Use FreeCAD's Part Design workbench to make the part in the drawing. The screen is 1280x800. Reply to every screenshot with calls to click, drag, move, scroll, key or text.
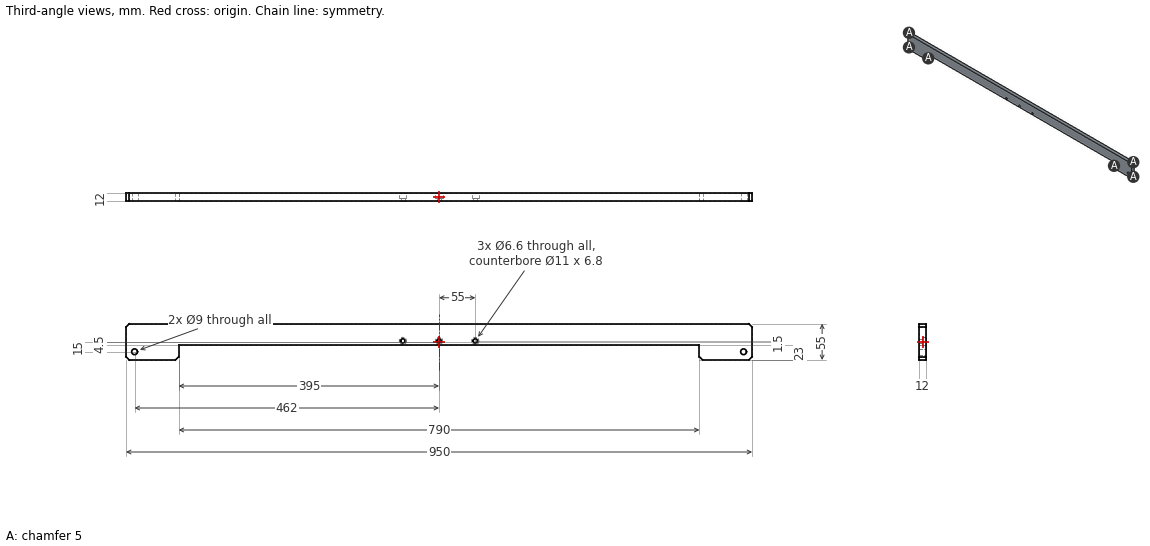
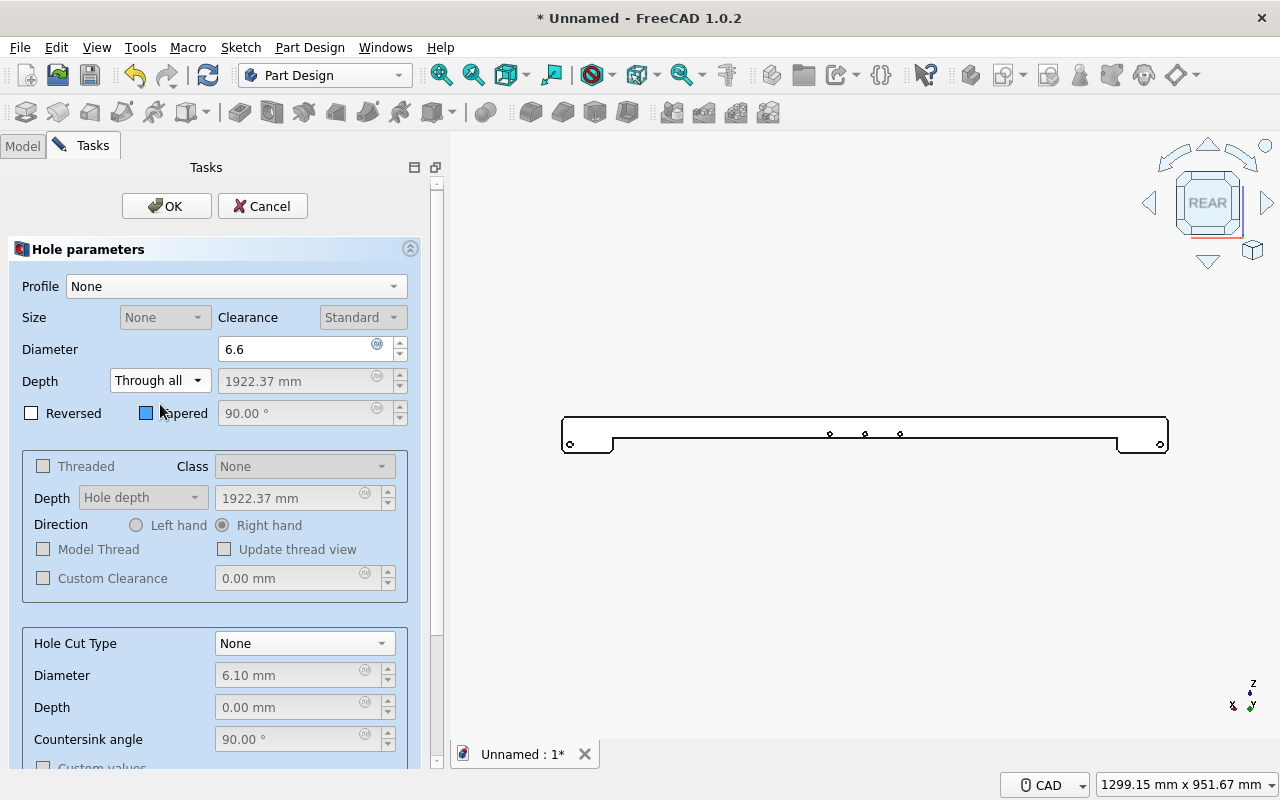
click(306, 644)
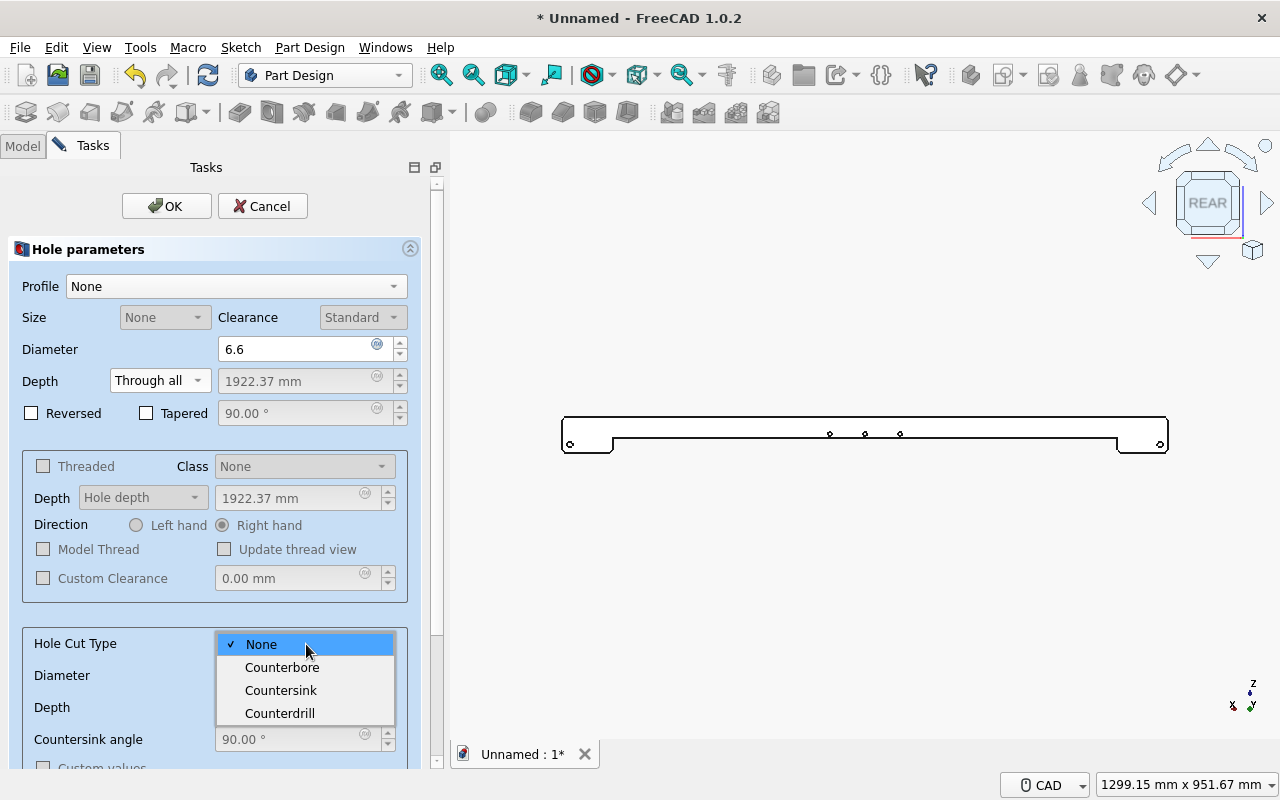
click(304, 668)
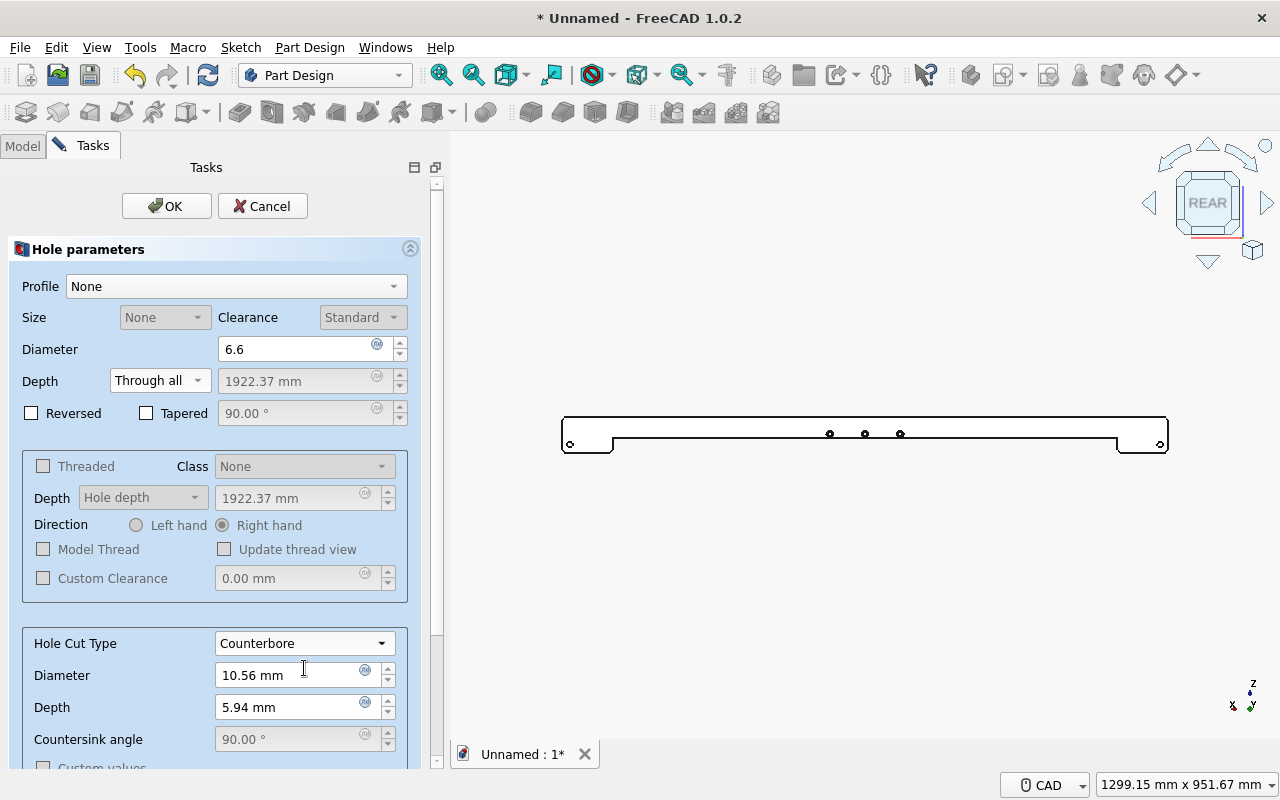
triple_click(298, 675)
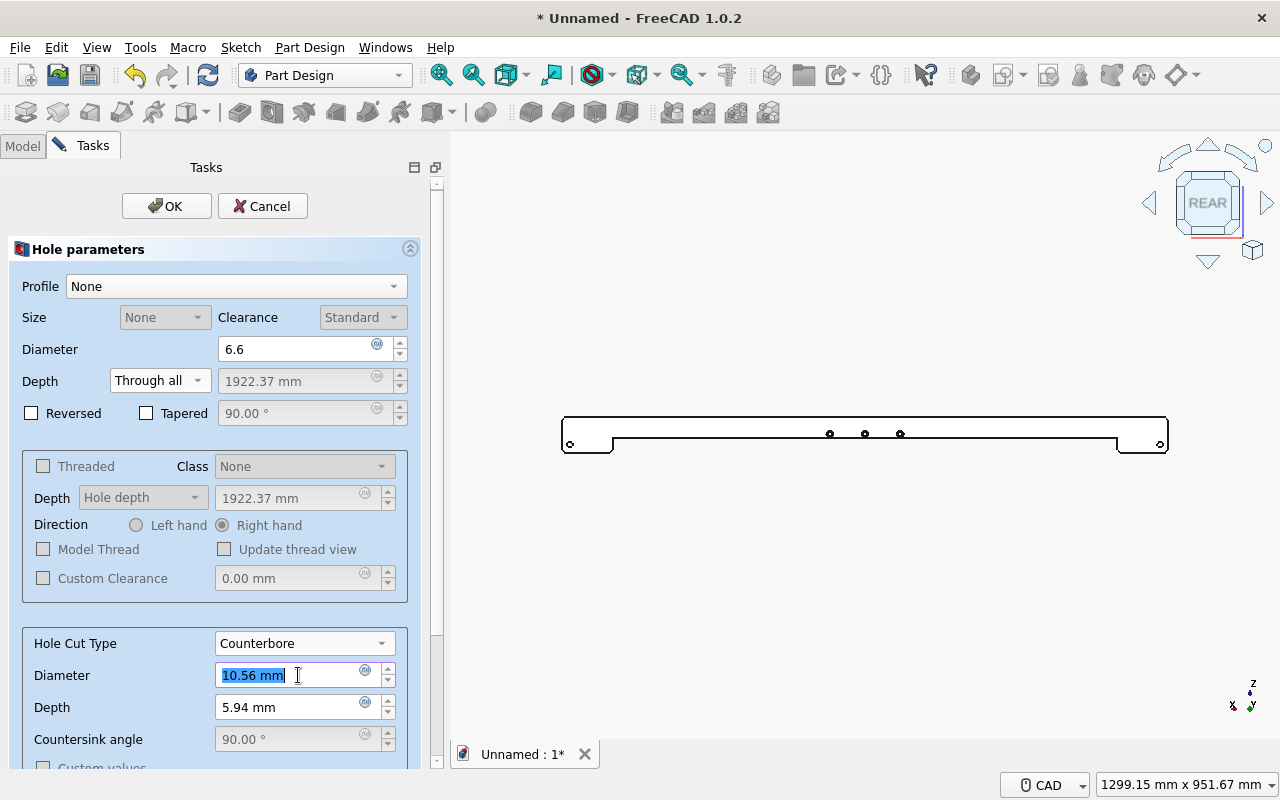
text(11)
key(Tab)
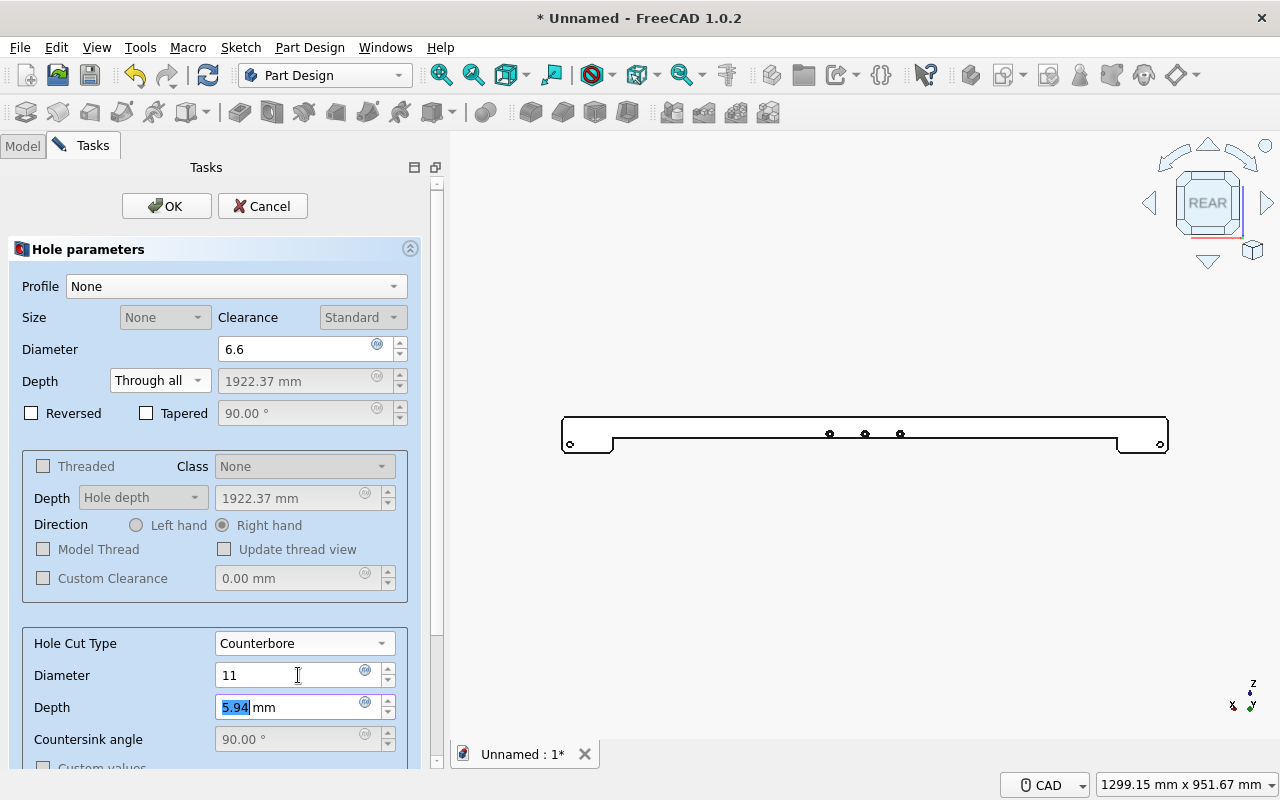
text(6.8)
key(Tab)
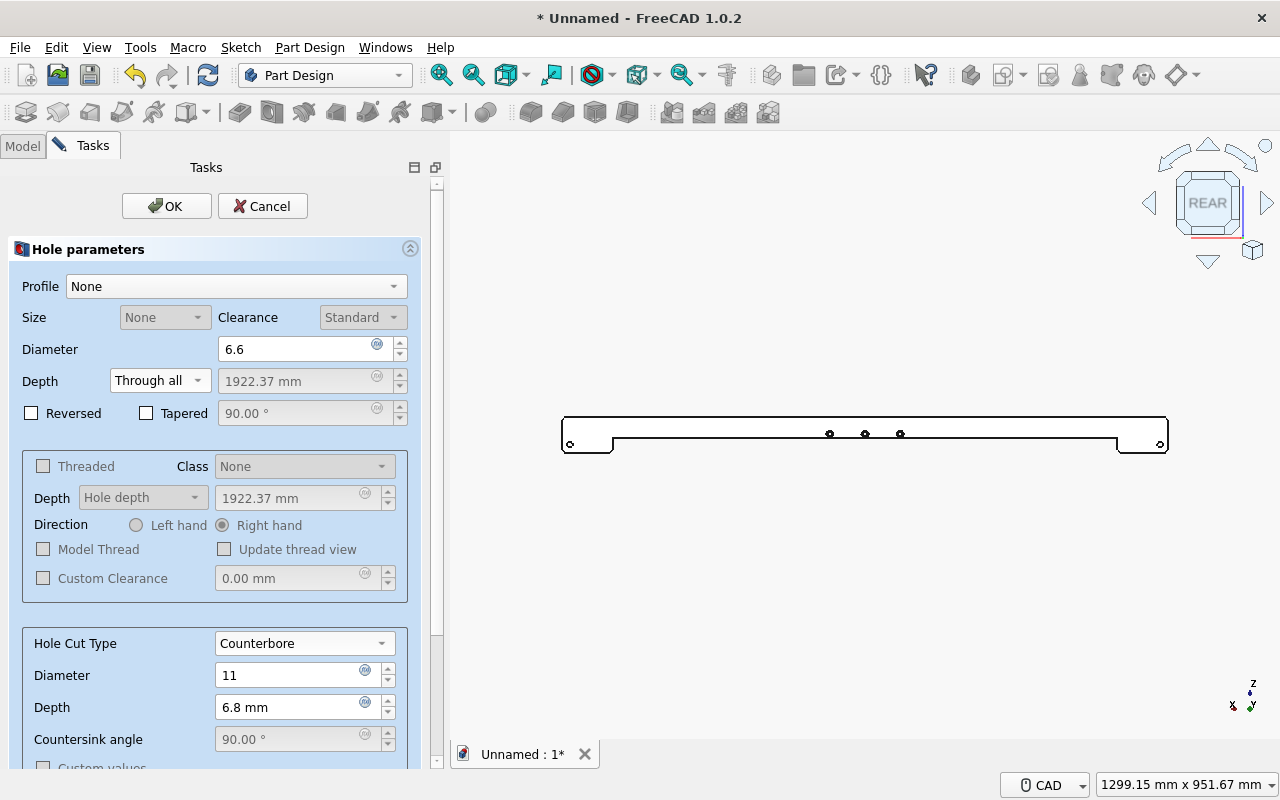
click(167, 206)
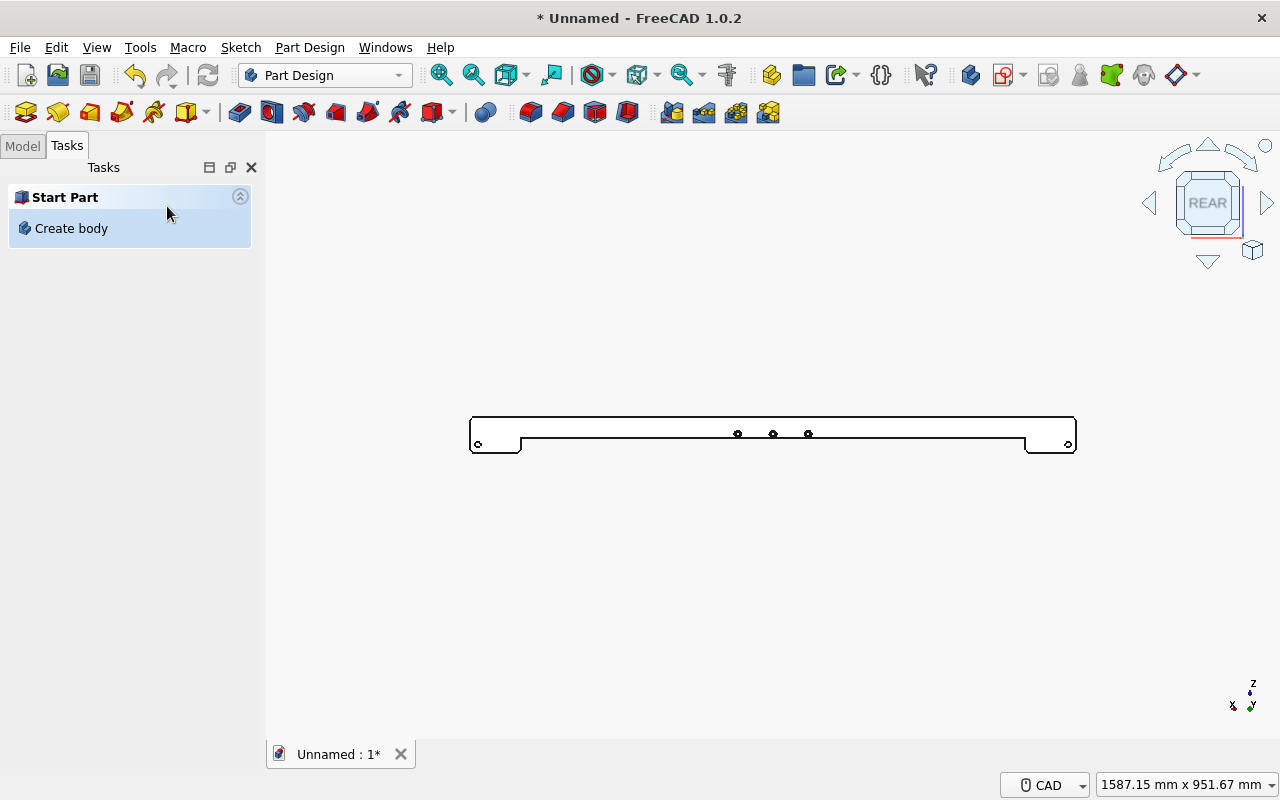
key(0)